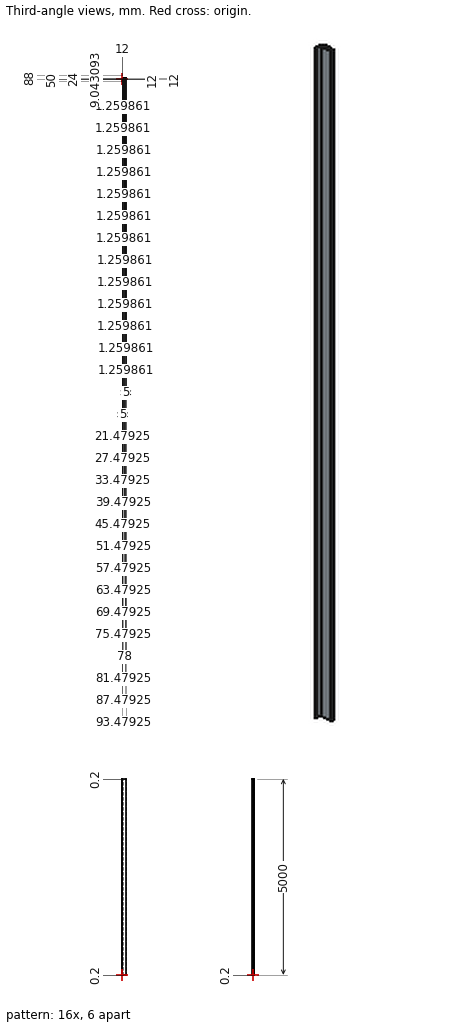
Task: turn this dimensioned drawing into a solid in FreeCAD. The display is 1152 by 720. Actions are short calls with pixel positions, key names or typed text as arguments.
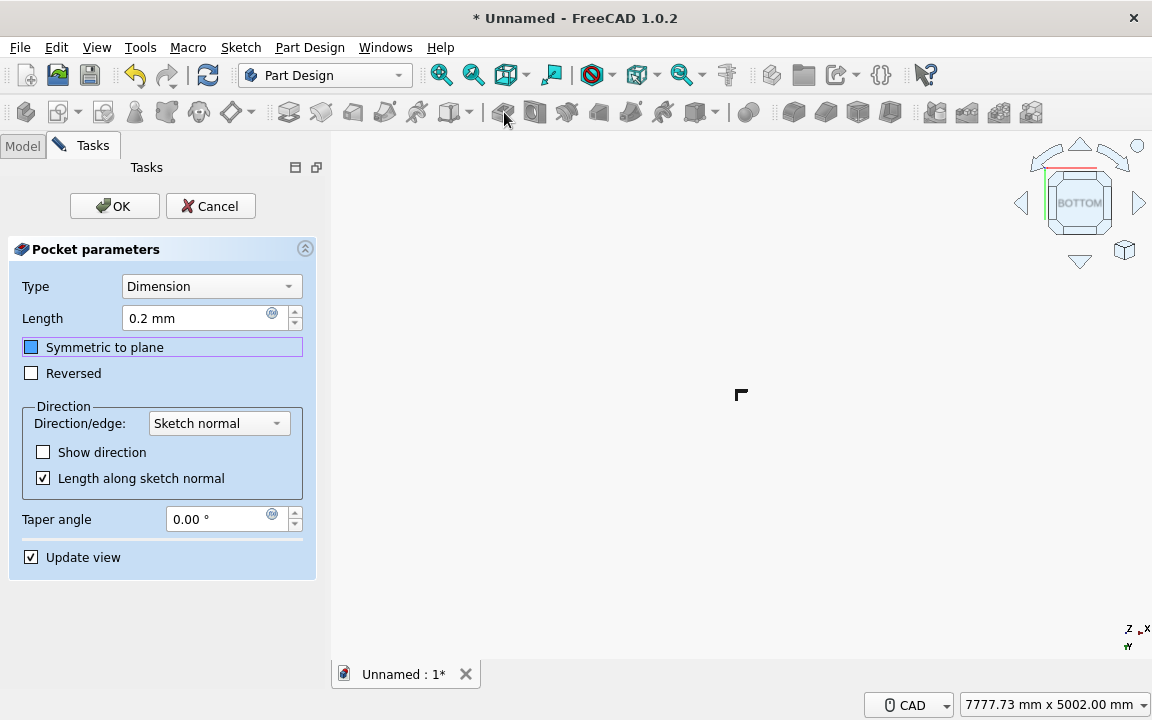
click(30, 373)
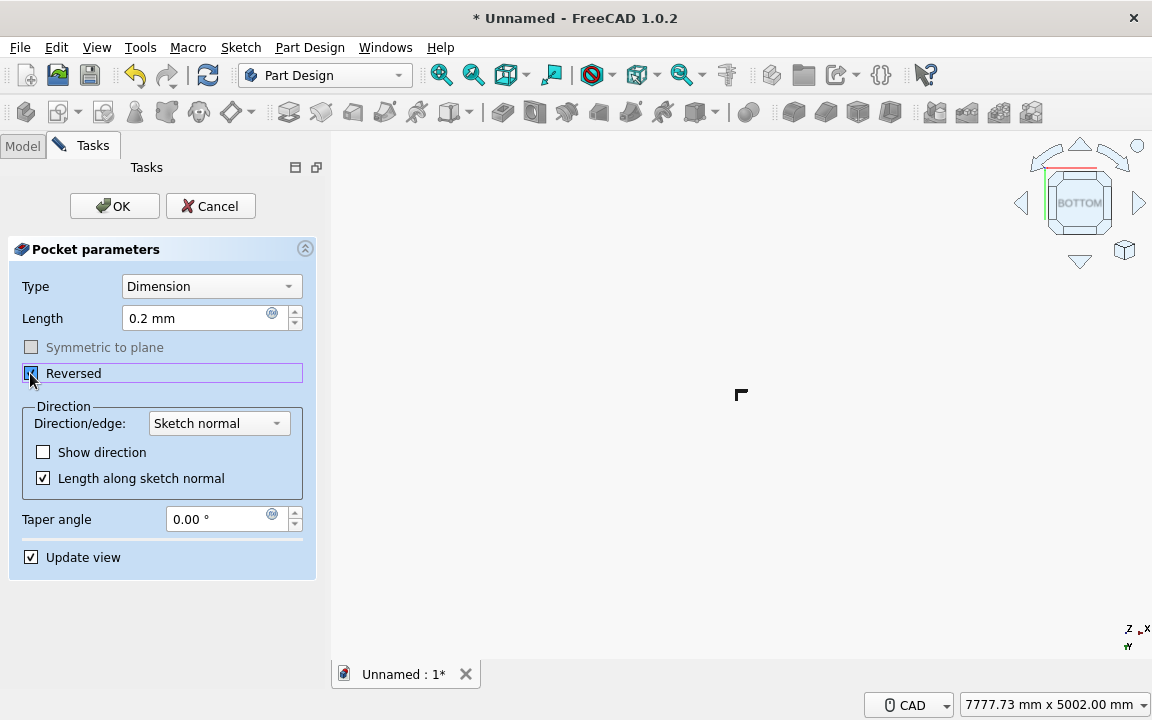
click(115, 206)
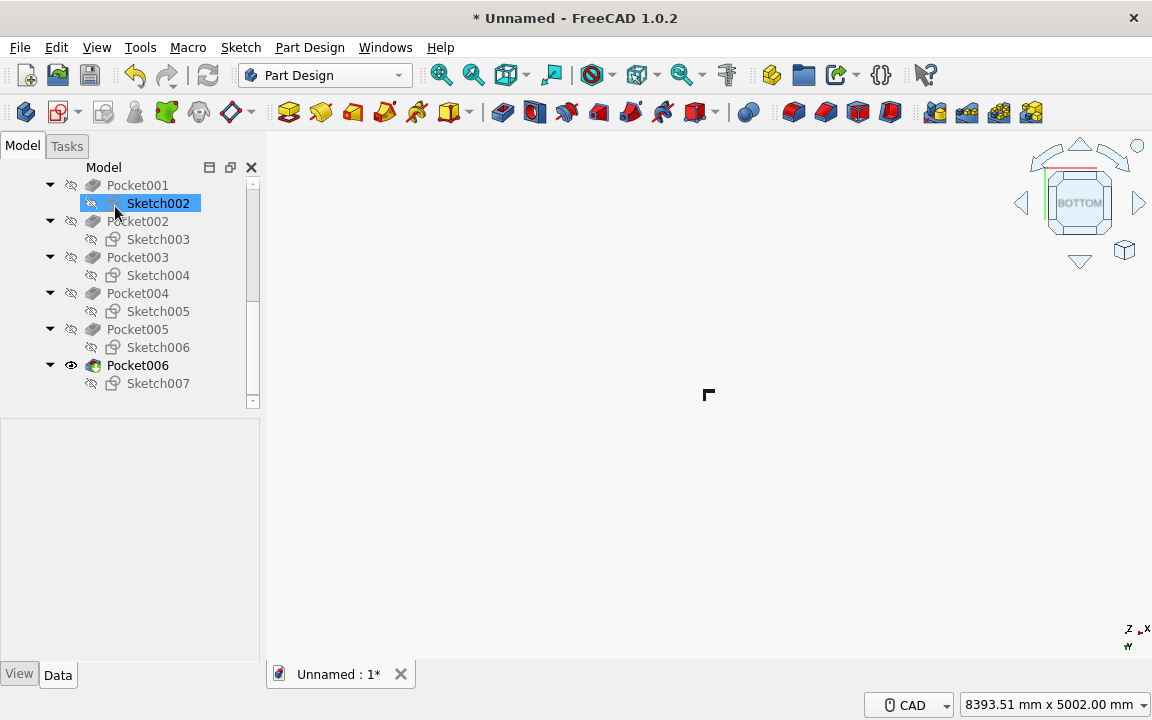
click(442, 76)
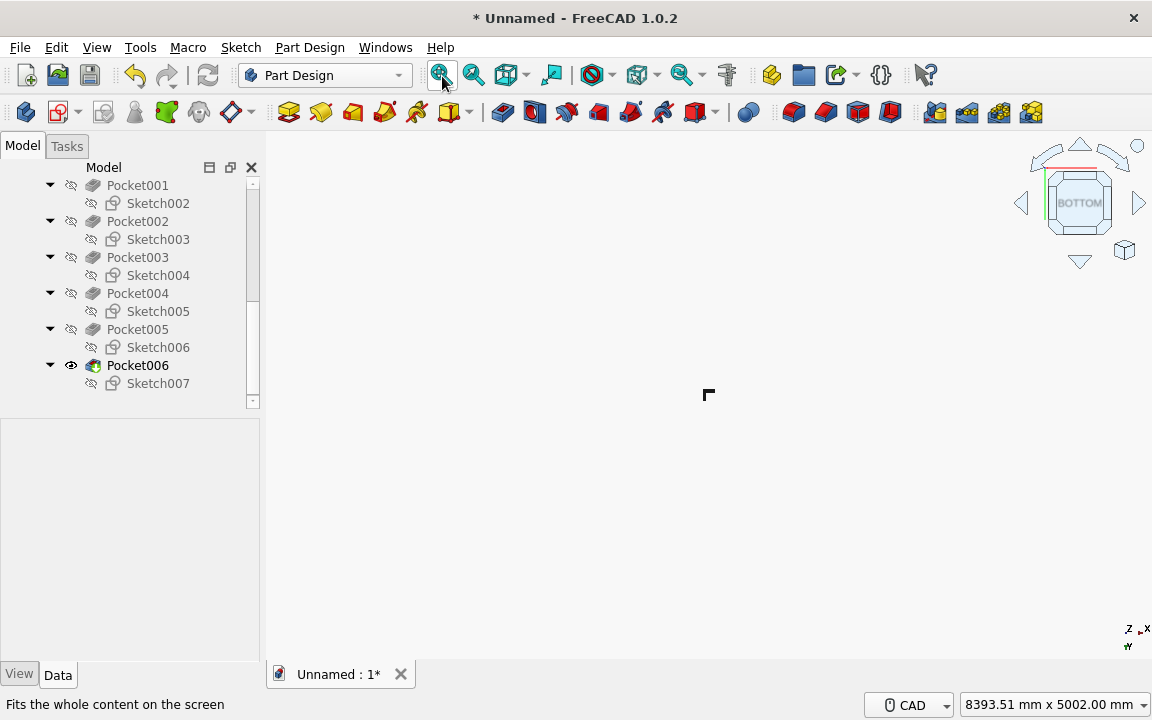
scroll(712, 389, up, 14)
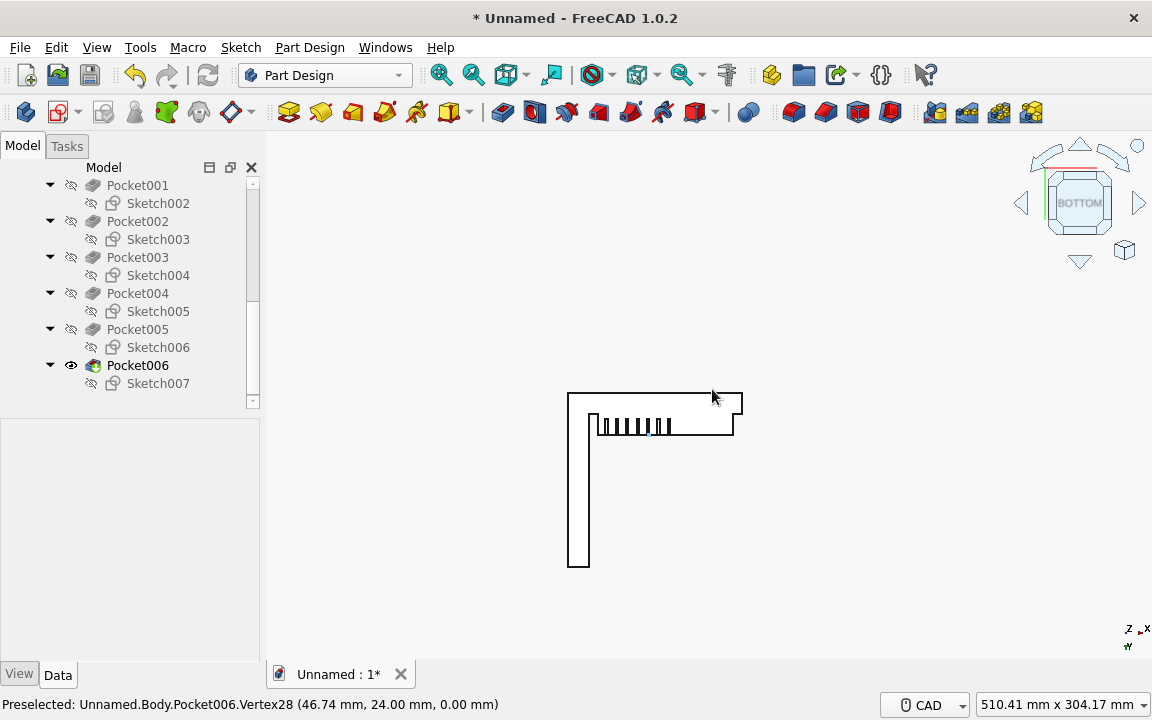
click(704, 405)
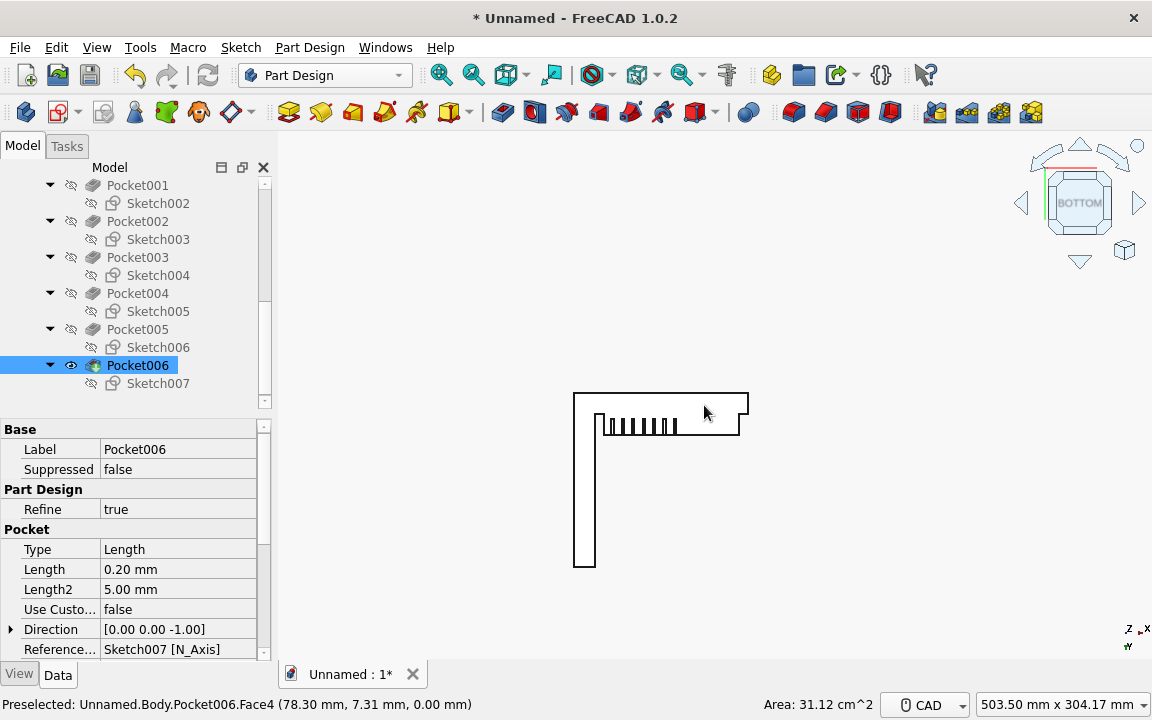
click(58, 112)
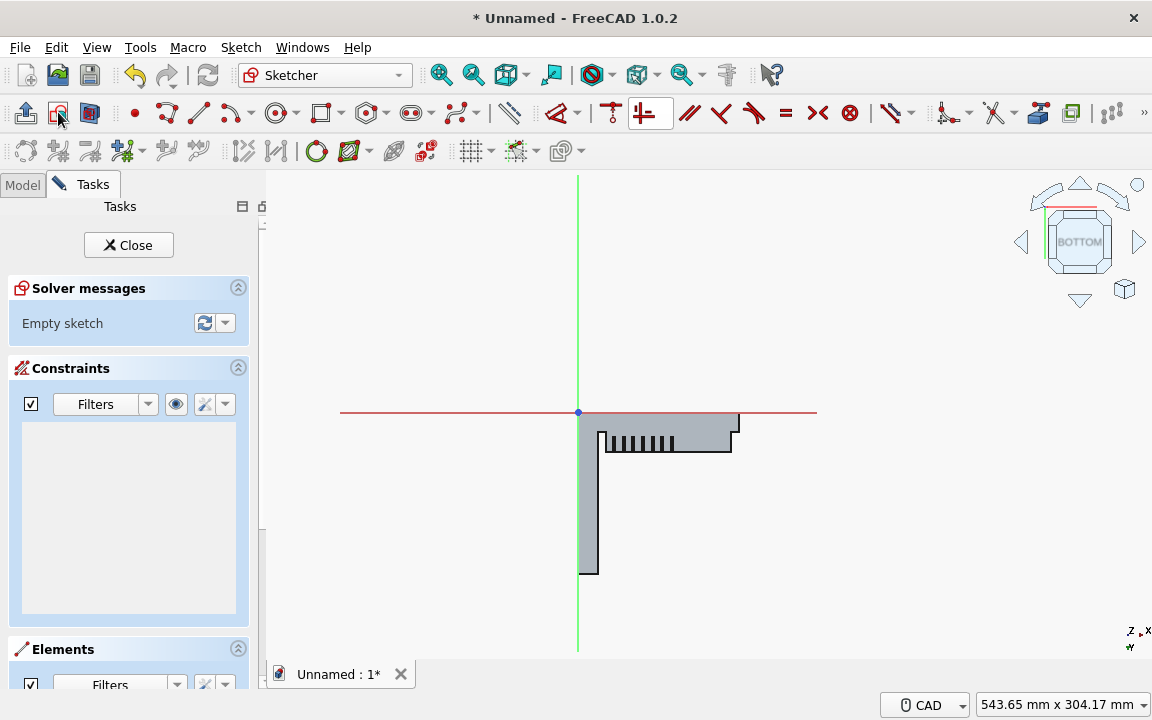
scroll(684, 446, up, 15)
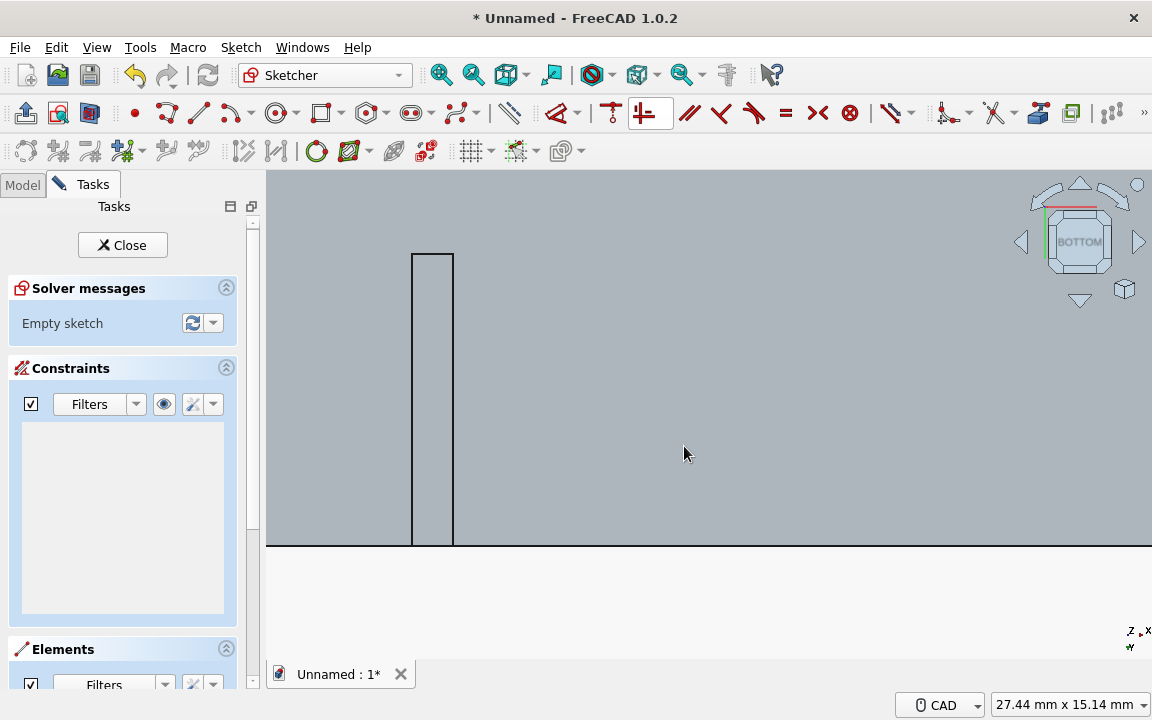
key(g)
key(r)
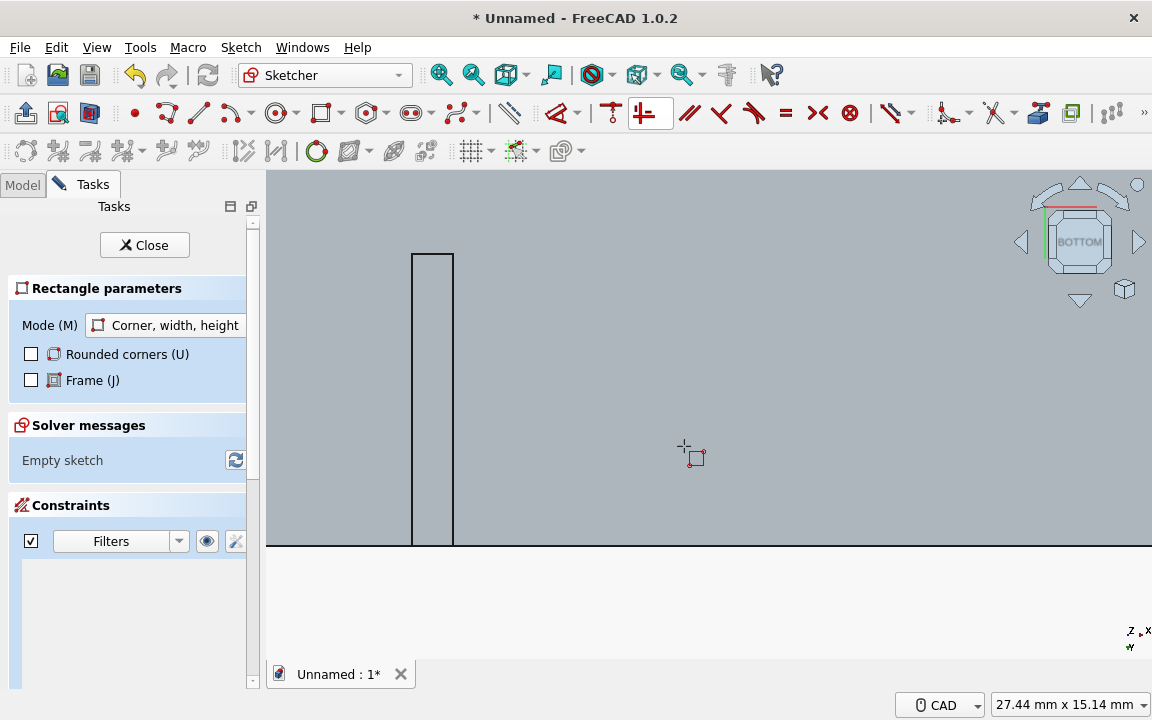
click(606, 254)
click(646, 546)
key(Escape)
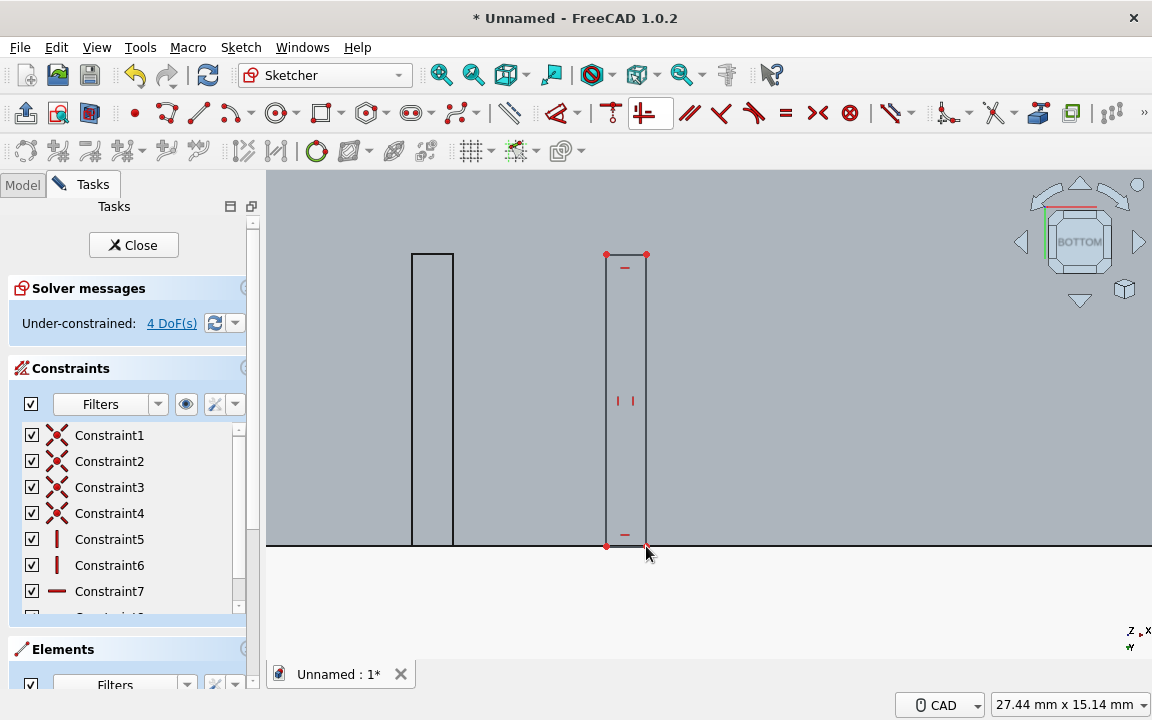
click(556, 114)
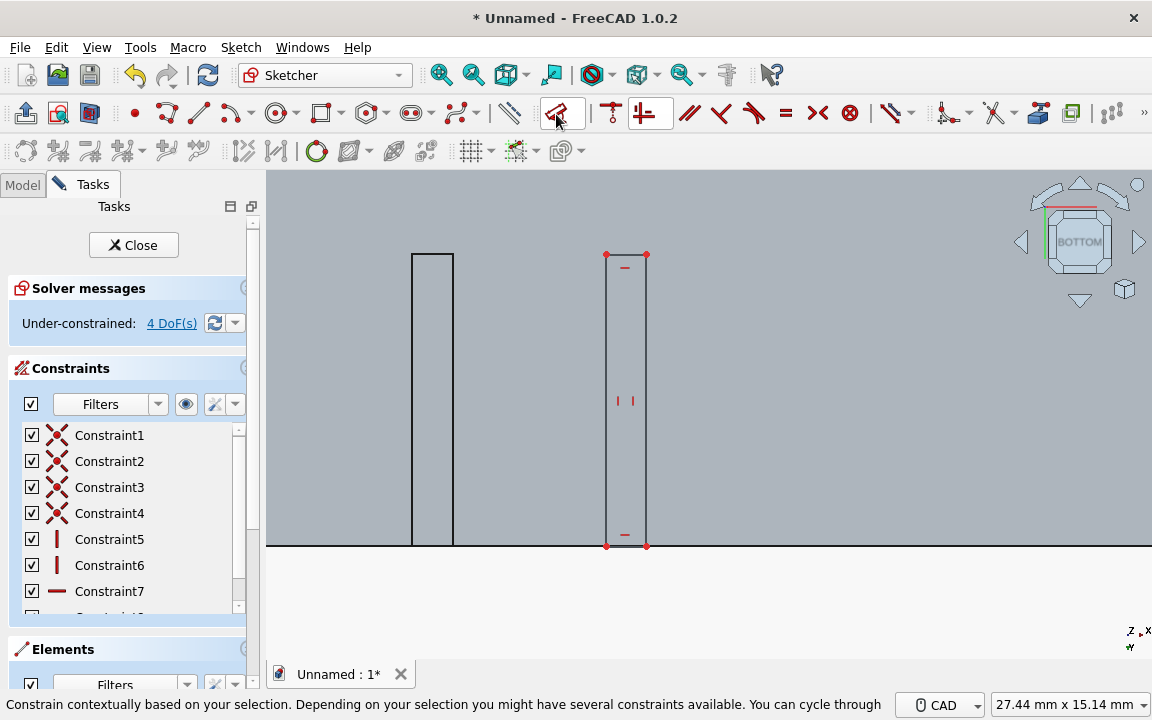
click(606, 547)
click(664, 373)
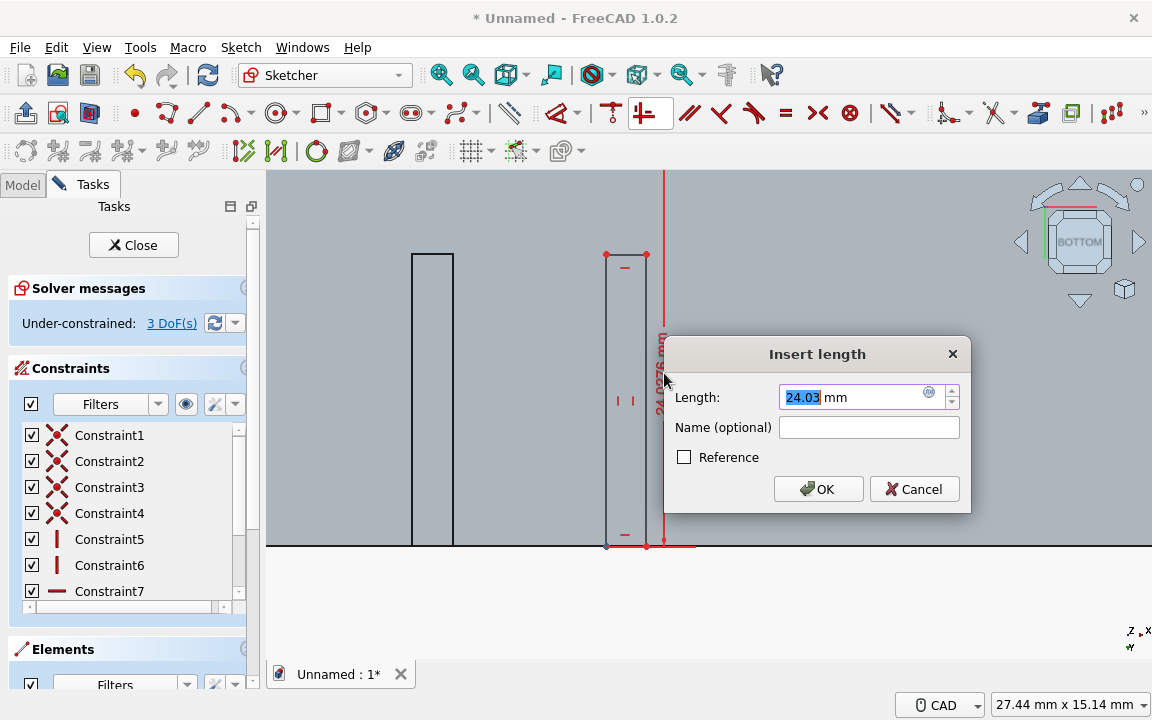
text(24)
key(Return)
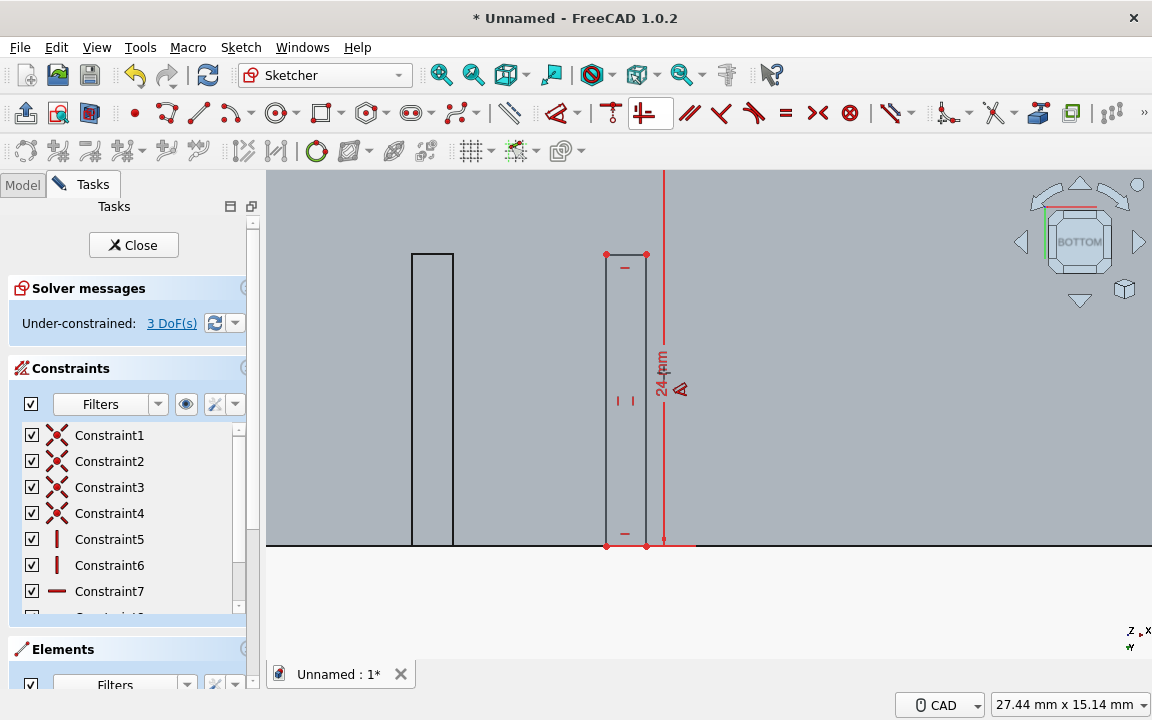
click(606, 342)
click(572, 401)